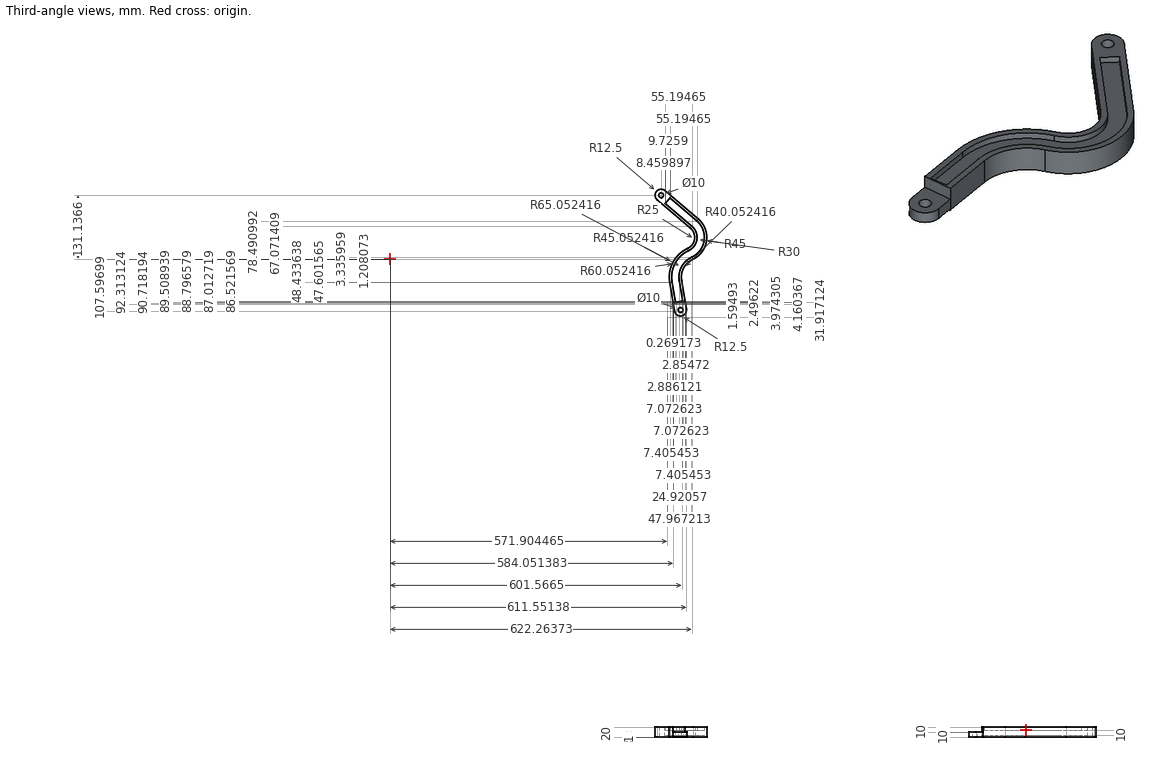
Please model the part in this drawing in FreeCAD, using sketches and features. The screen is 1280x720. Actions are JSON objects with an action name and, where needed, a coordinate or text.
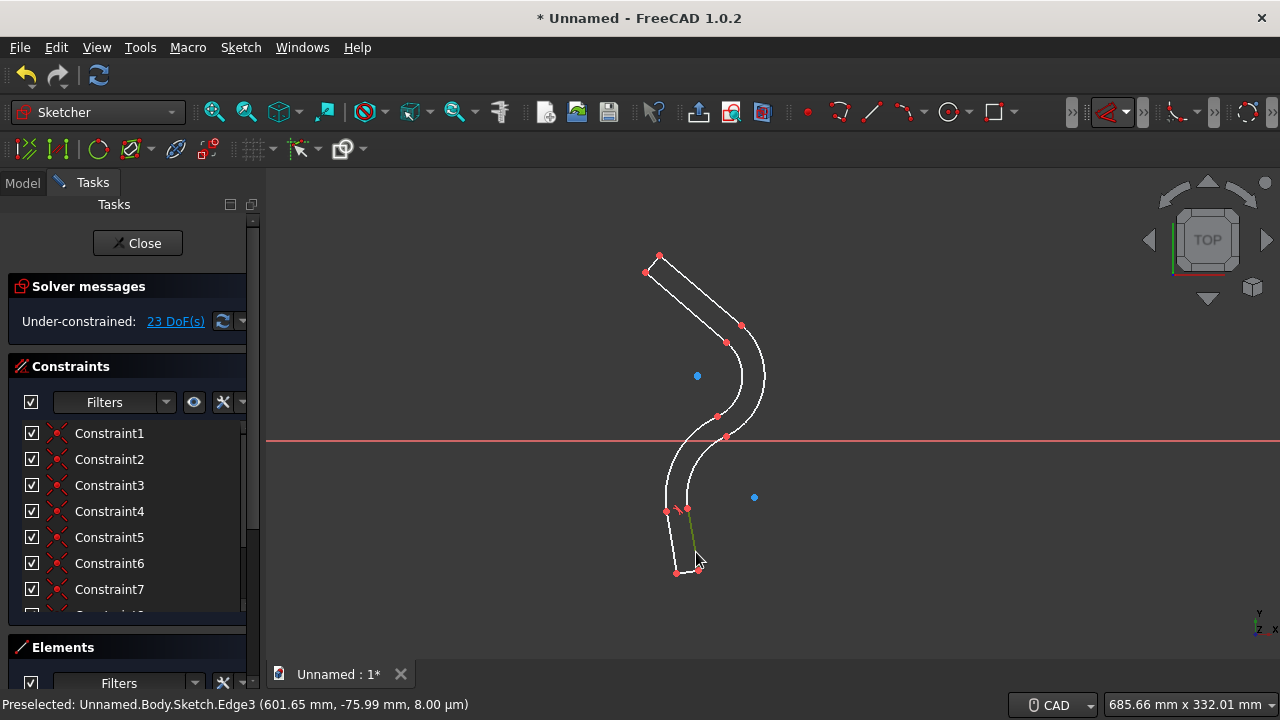
{"action": "scroll", "coordinate": [705, 451], "scroll_direction": "up", "scroll_amount": 2}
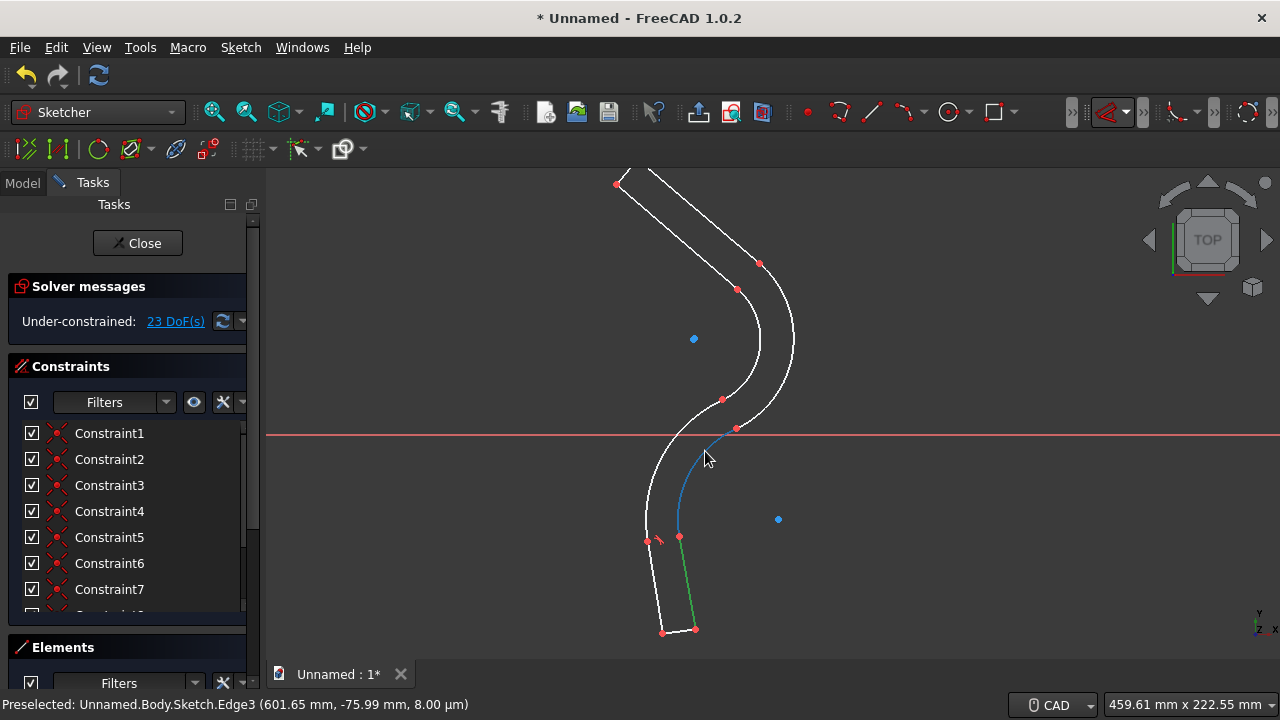
{"action": "left_click", "coordinate": [705, 451]}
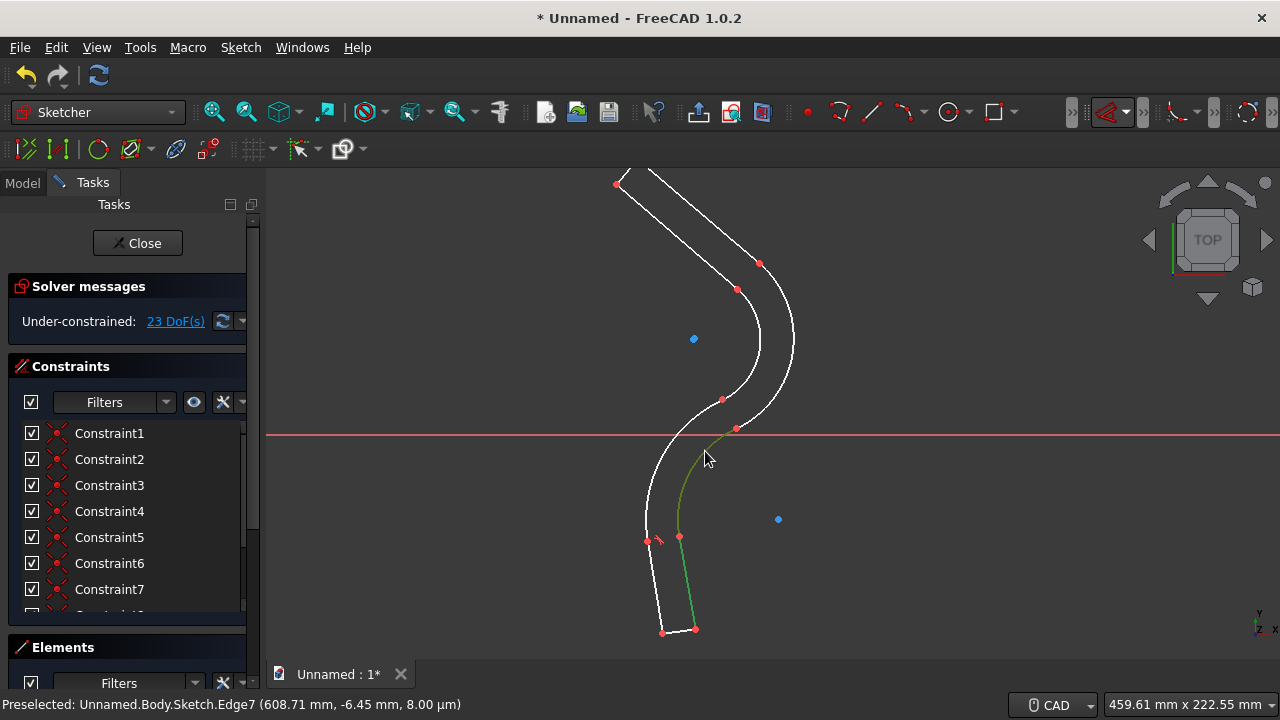
{"action": "key", "text": "t"}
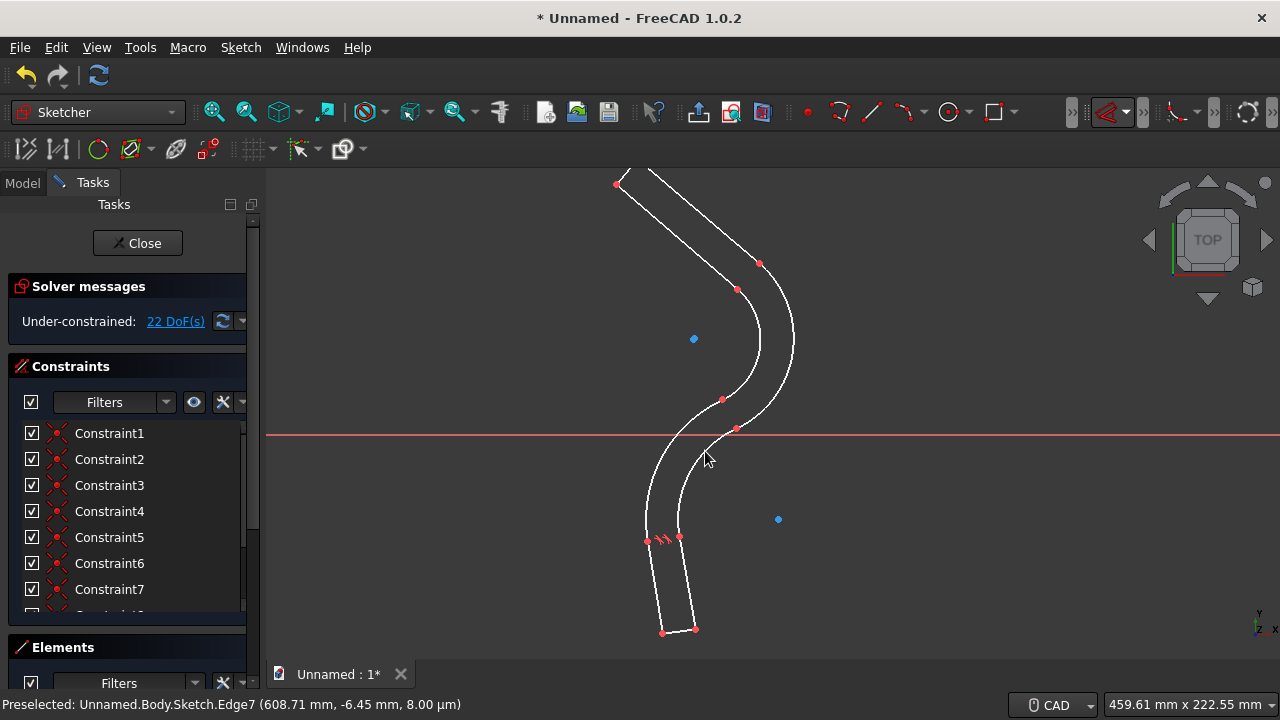
{"action": "left_click", "coordinate": [723, 232]}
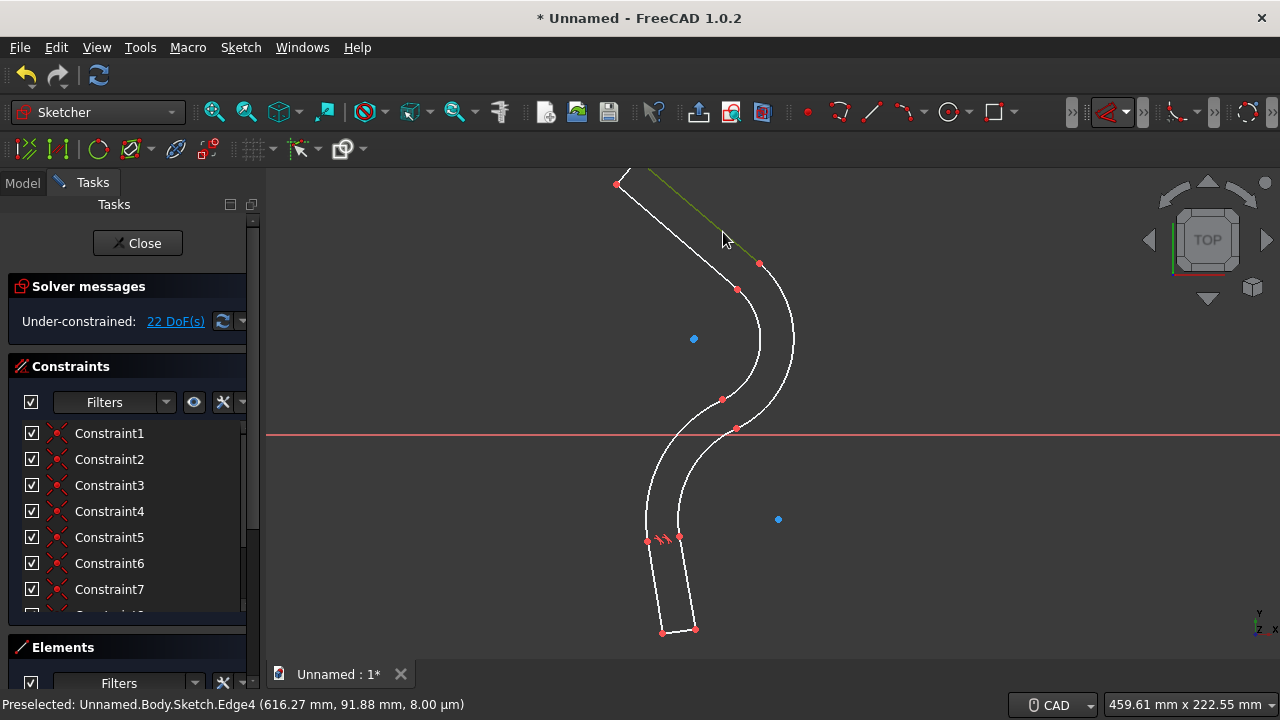
{"action": "left_click", "coordinate": [780, 389]}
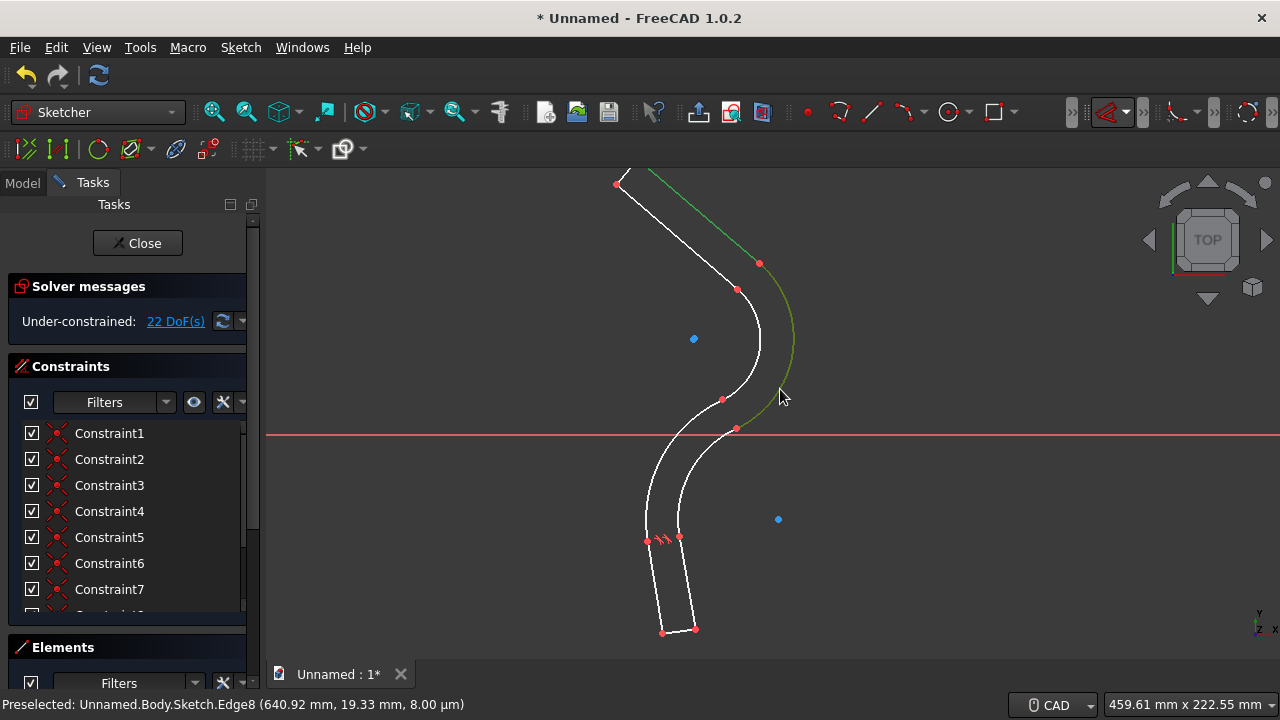
{"action": "key", "text": "t"}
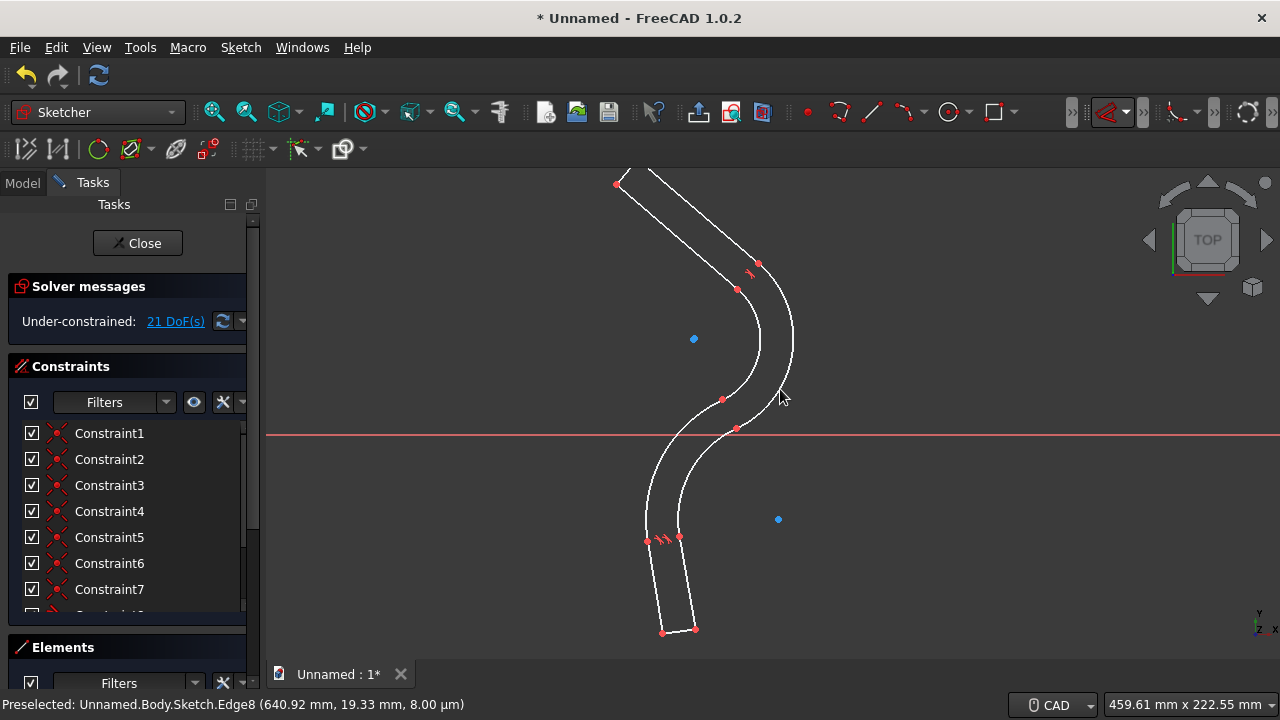
{"action": "left_click", "coordinate": [653, 216]}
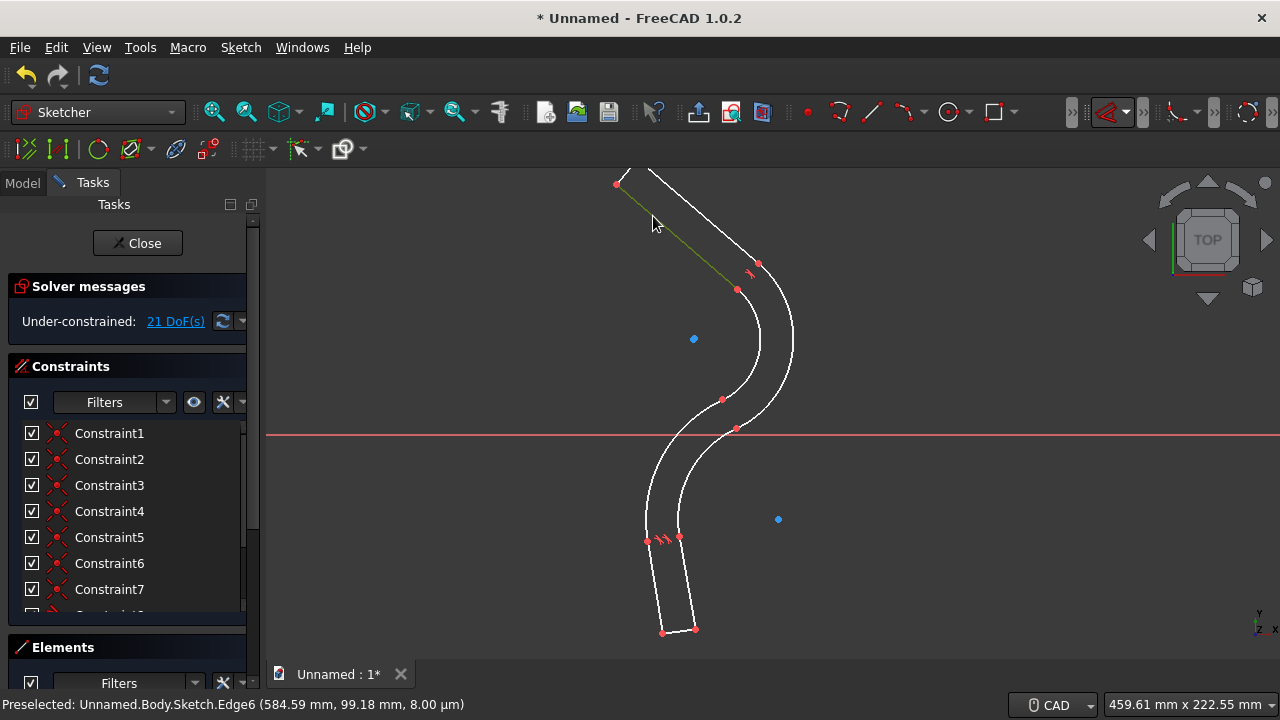
{"action": "left_click", "coordinate": [751, 373]}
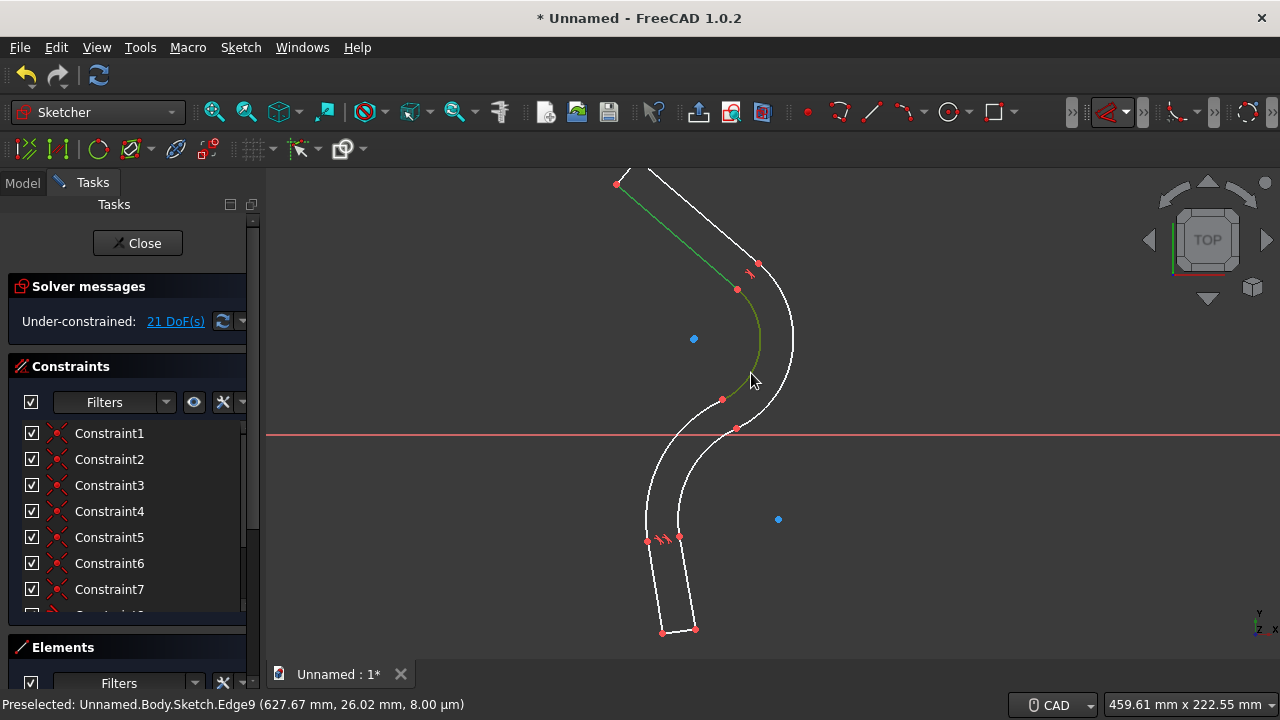
{"action": "key", "text": "t"}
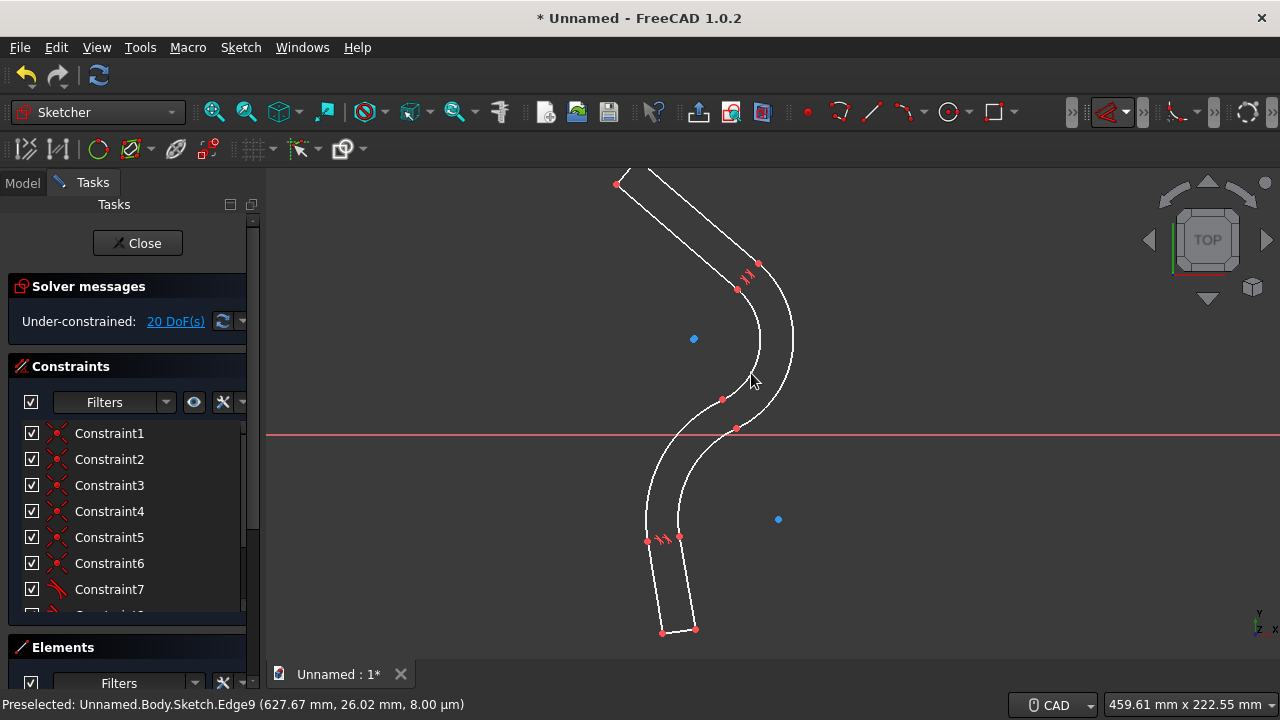
{"action": "left_click", "coordinate": [705, 451]}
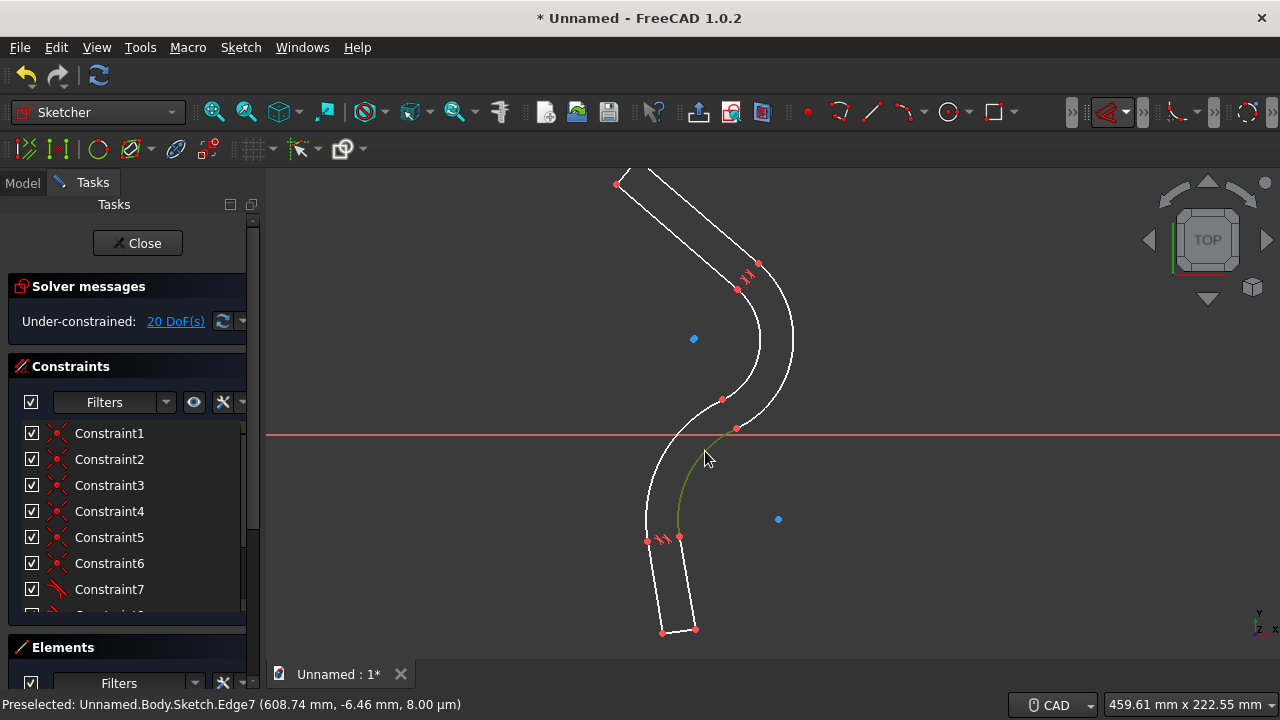
{"action": "left_click", "coordinate": [780, 389]}